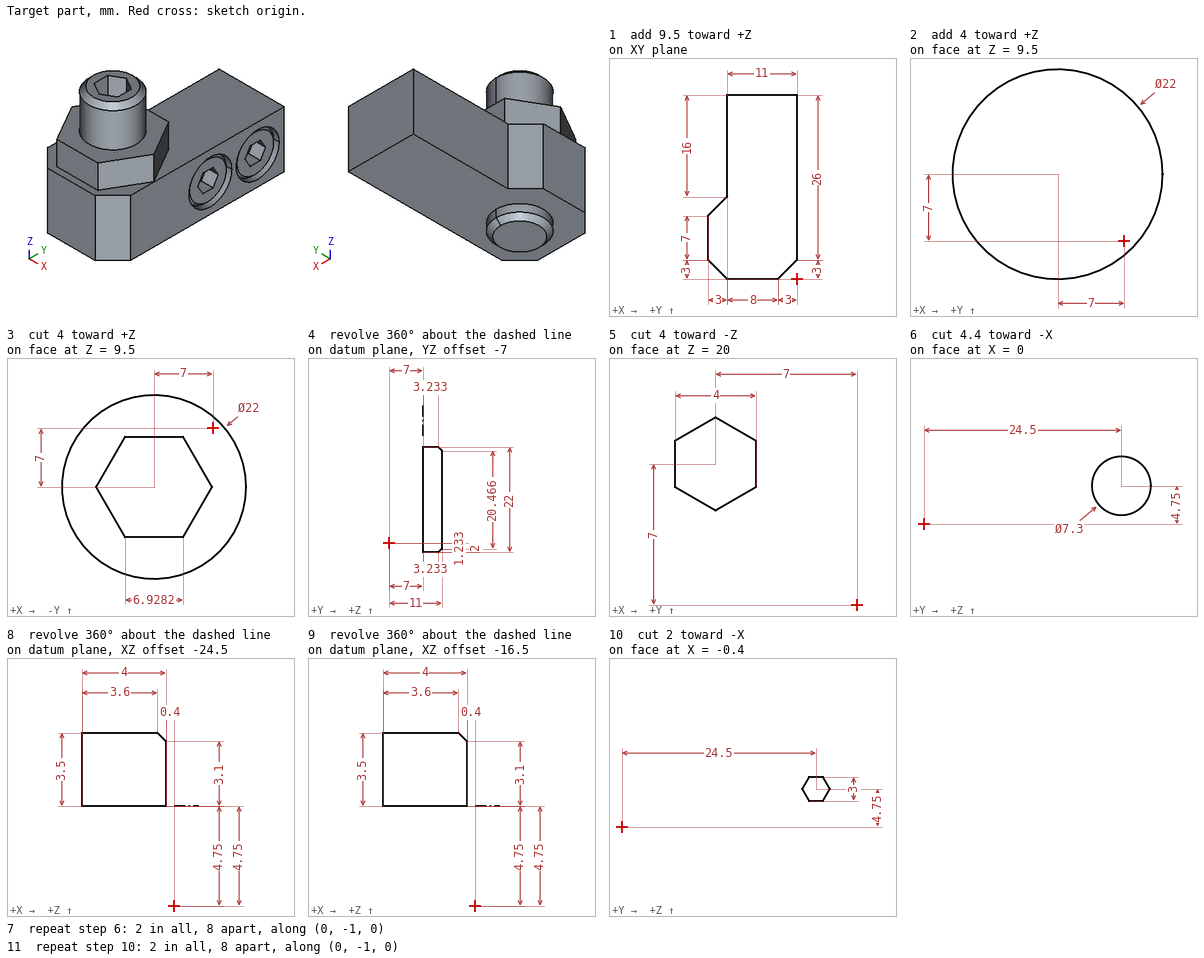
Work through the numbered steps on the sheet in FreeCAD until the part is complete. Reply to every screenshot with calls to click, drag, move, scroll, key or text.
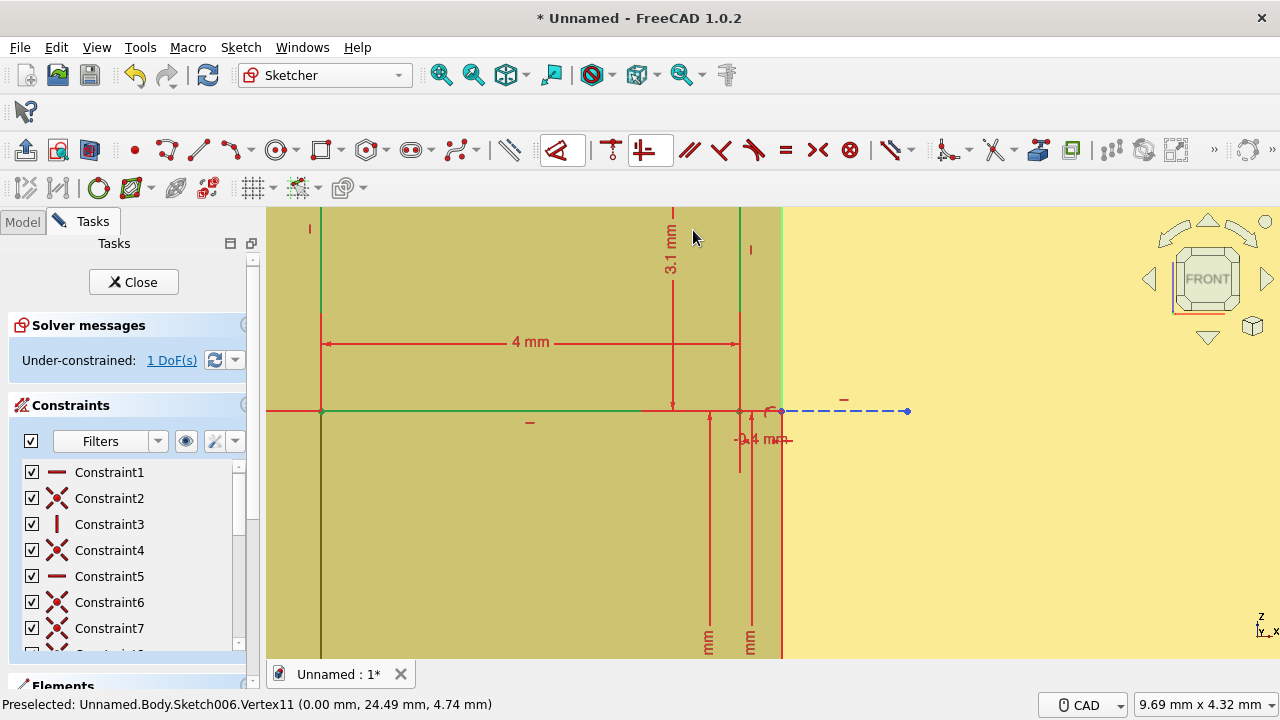
click(134, 282)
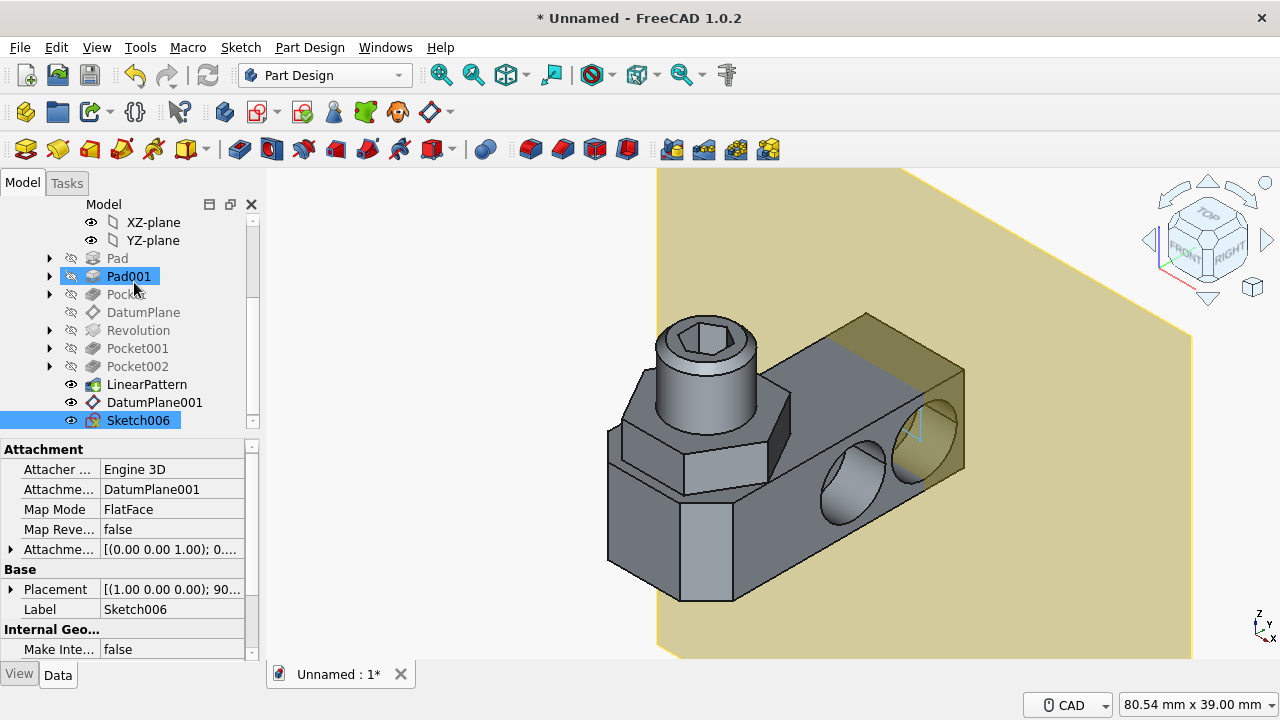
click(58, 150)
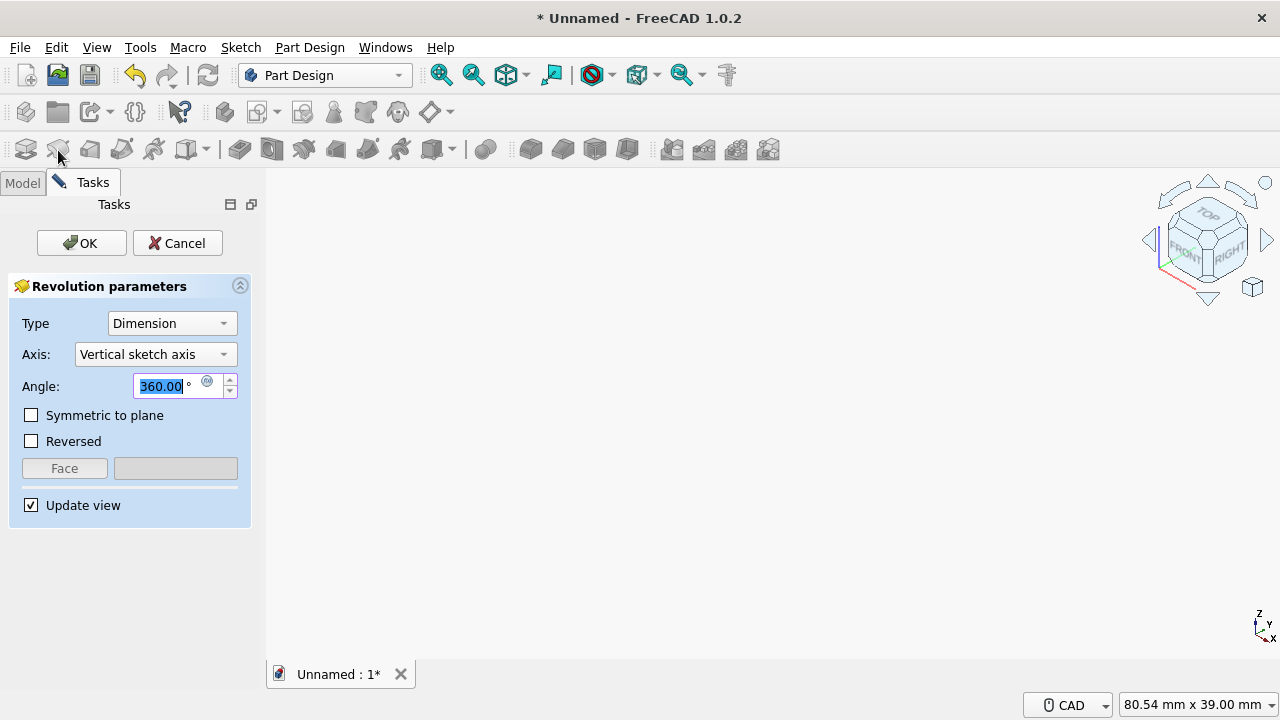
click(156, 354)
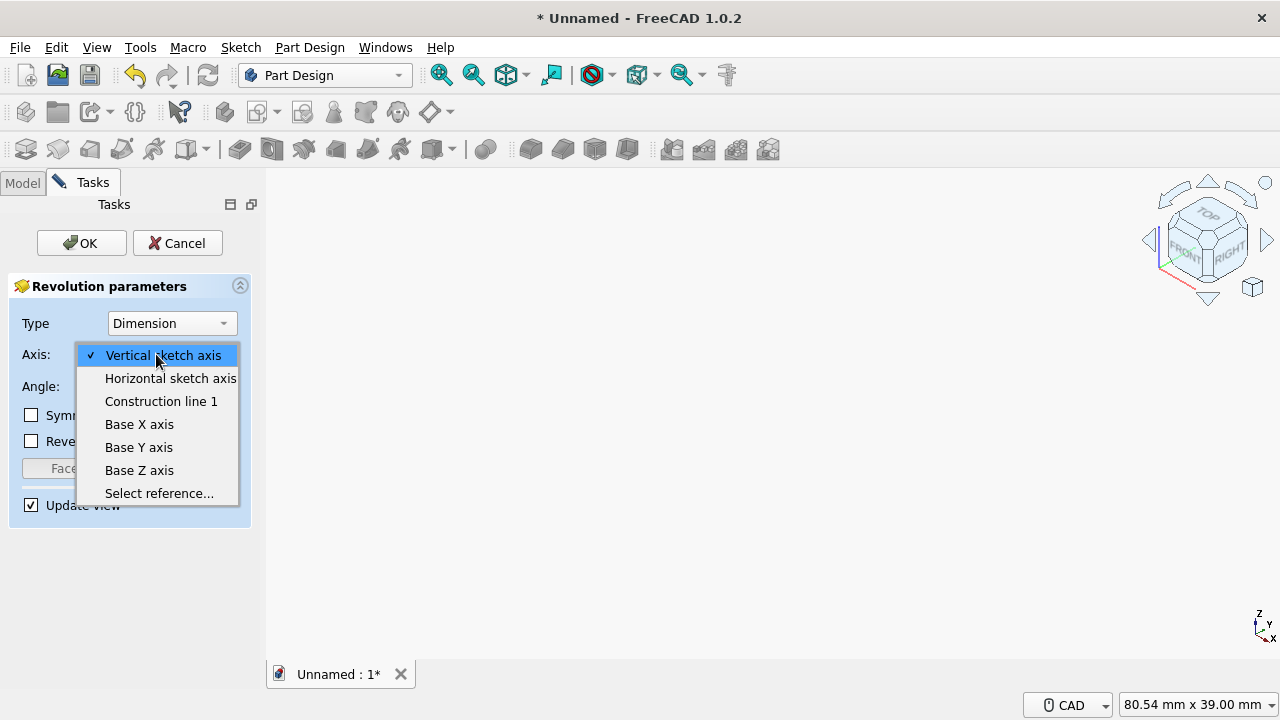
click(156, 402)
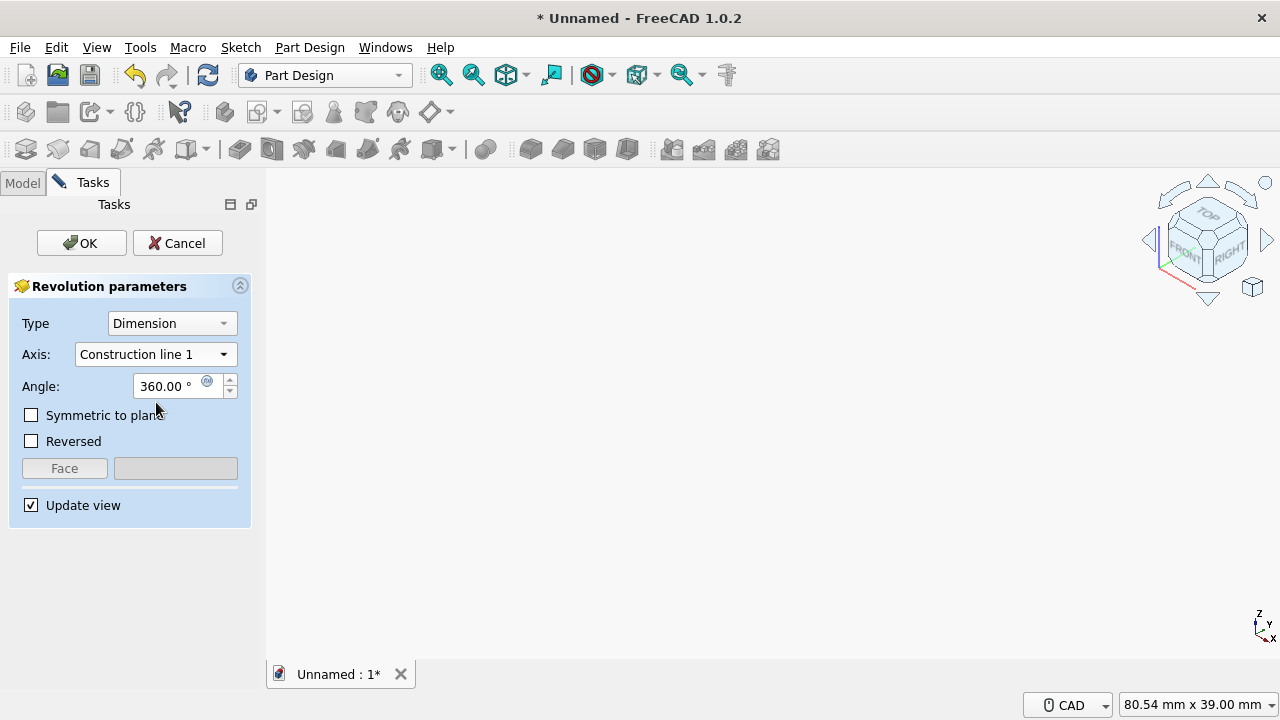
click(82, 243)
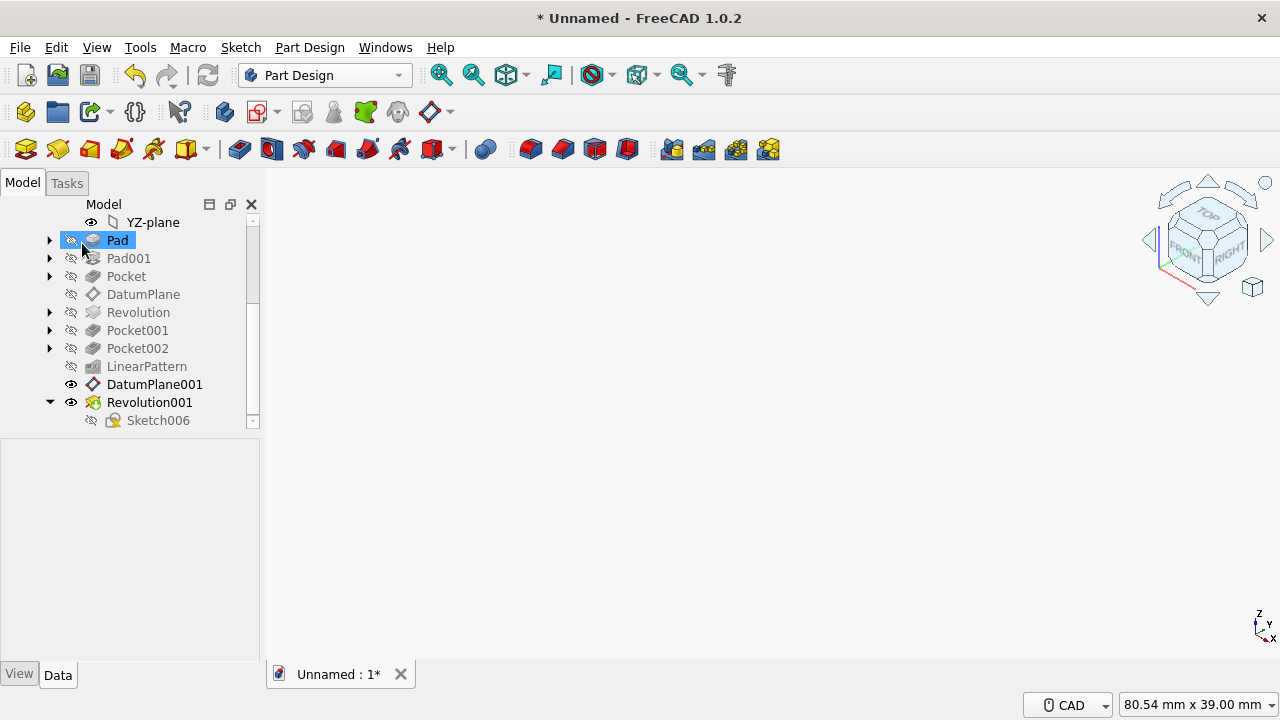
click(116, 384)
key(space)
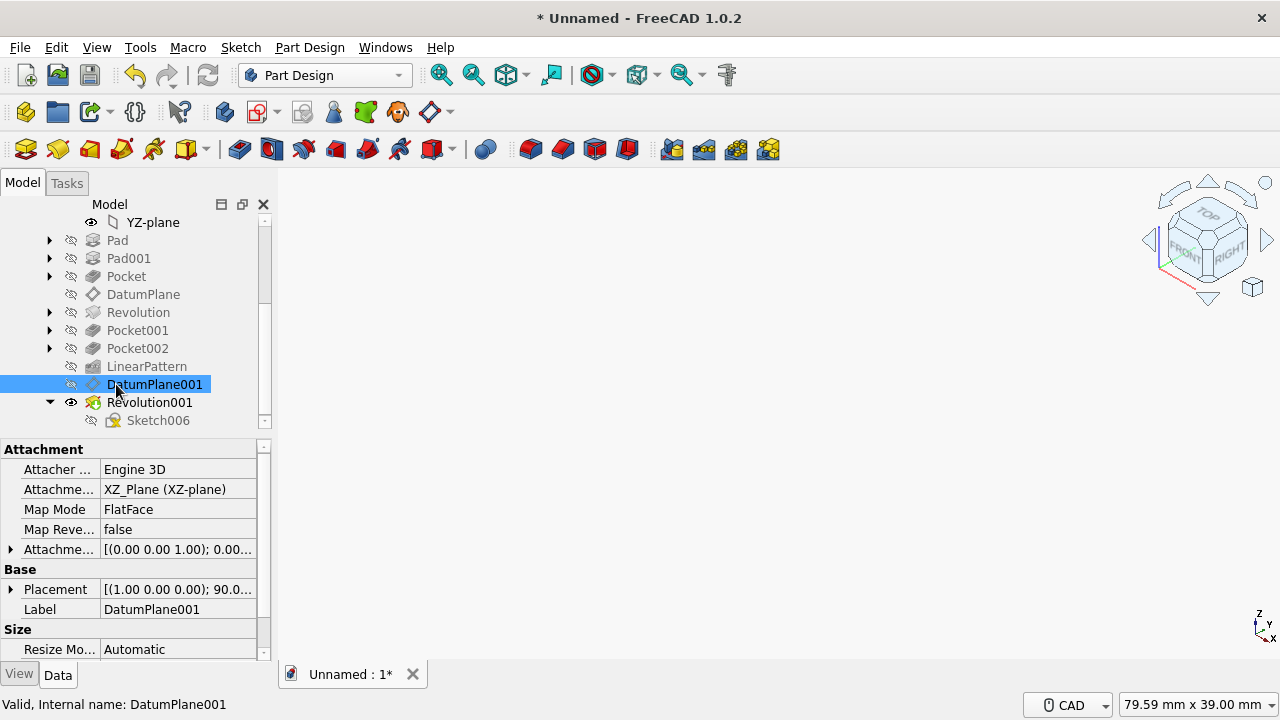
key(v)
key(f)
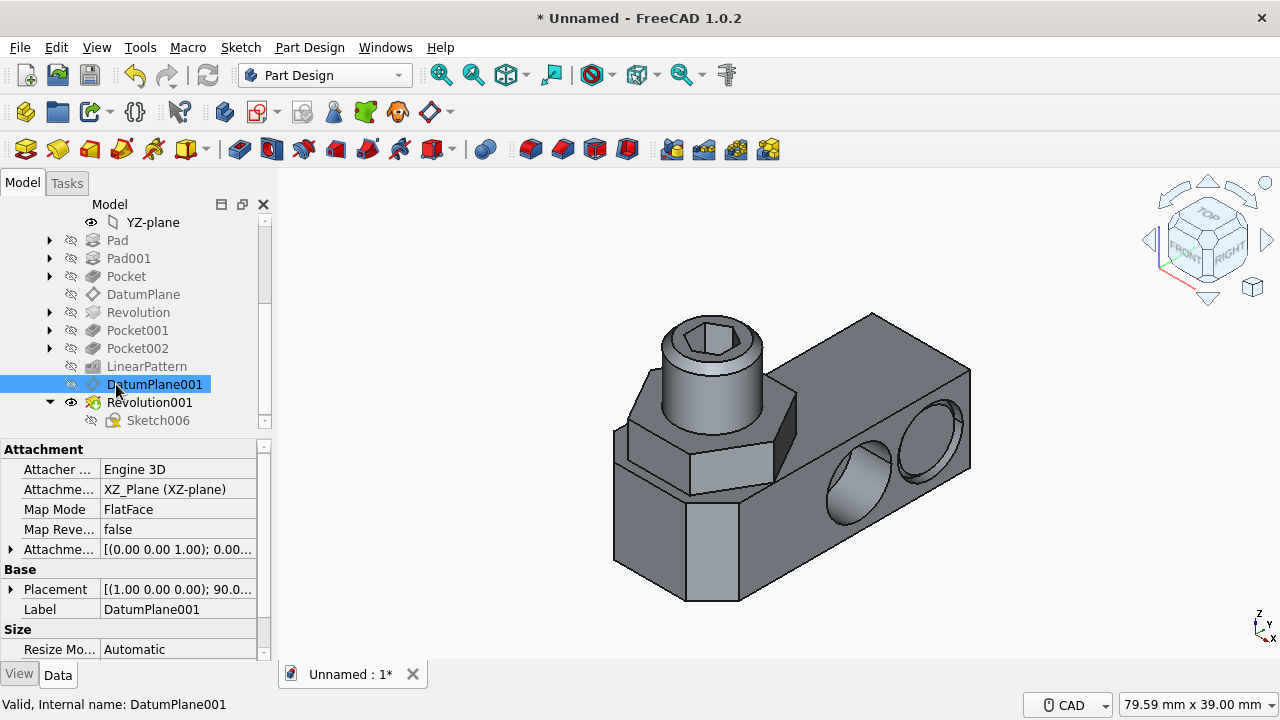
scroll(160, 326, down, 3)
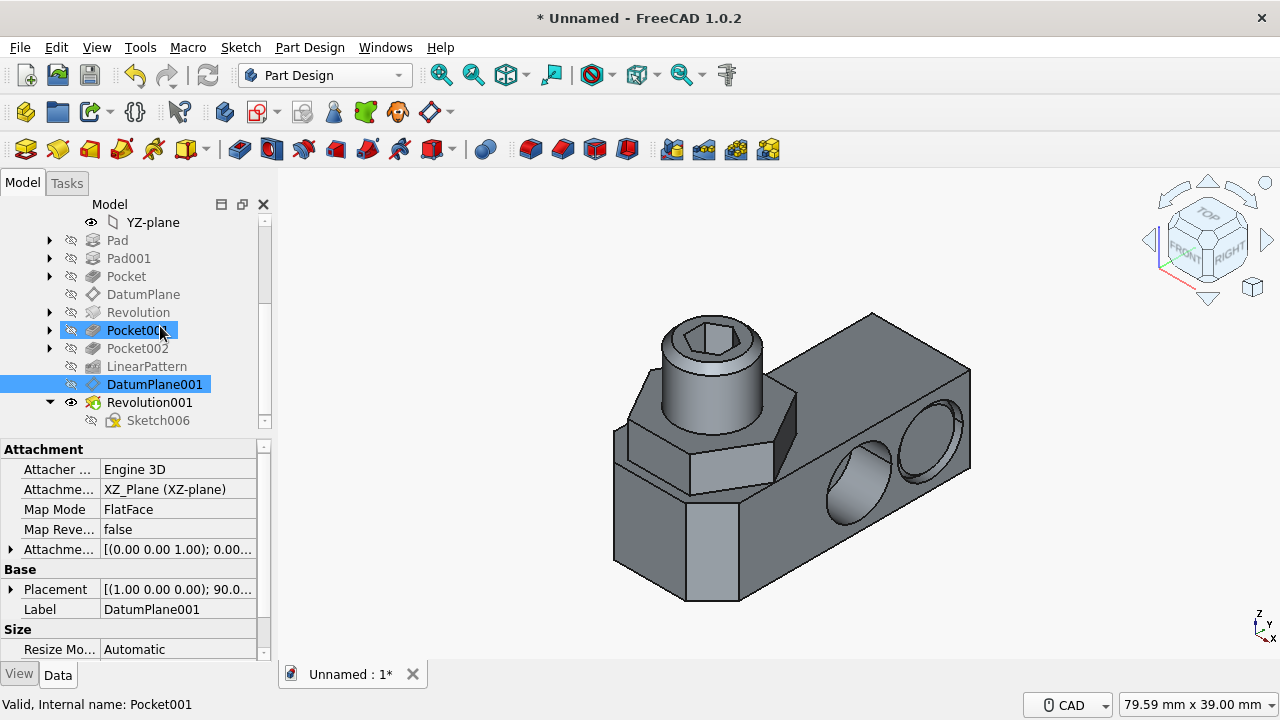
scroll(160, 326, up, 15)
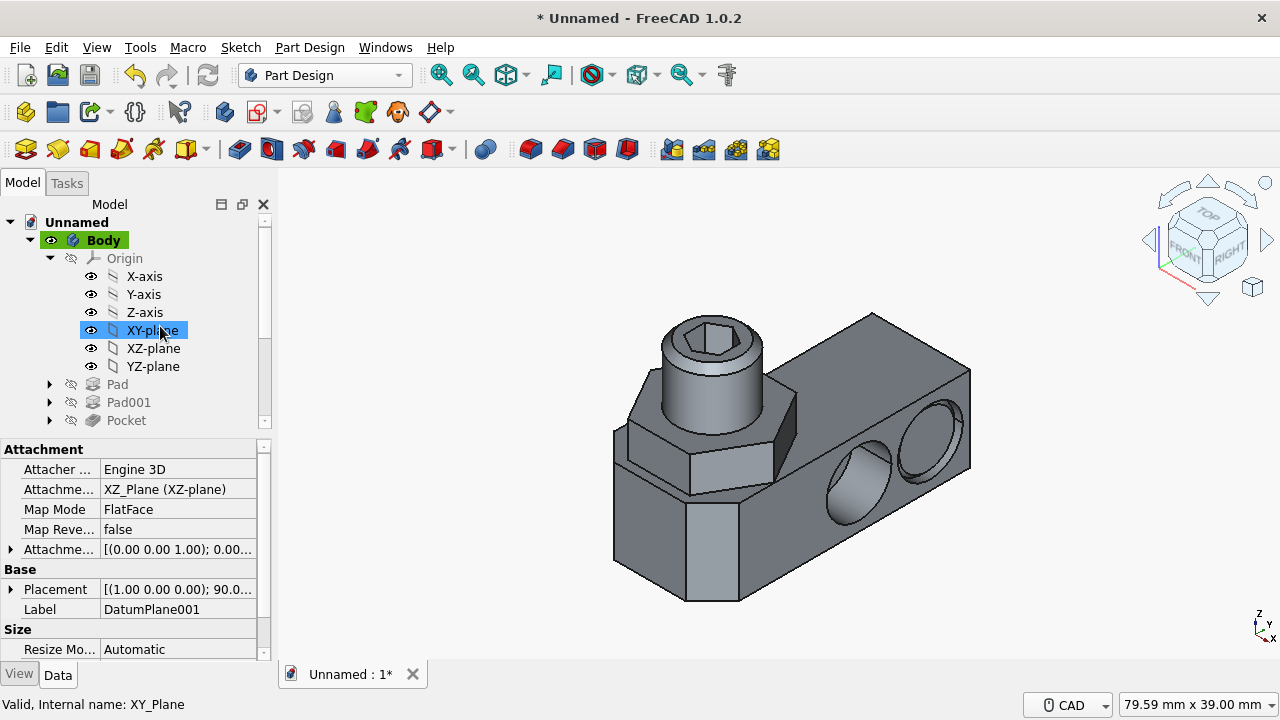
click(136, 348)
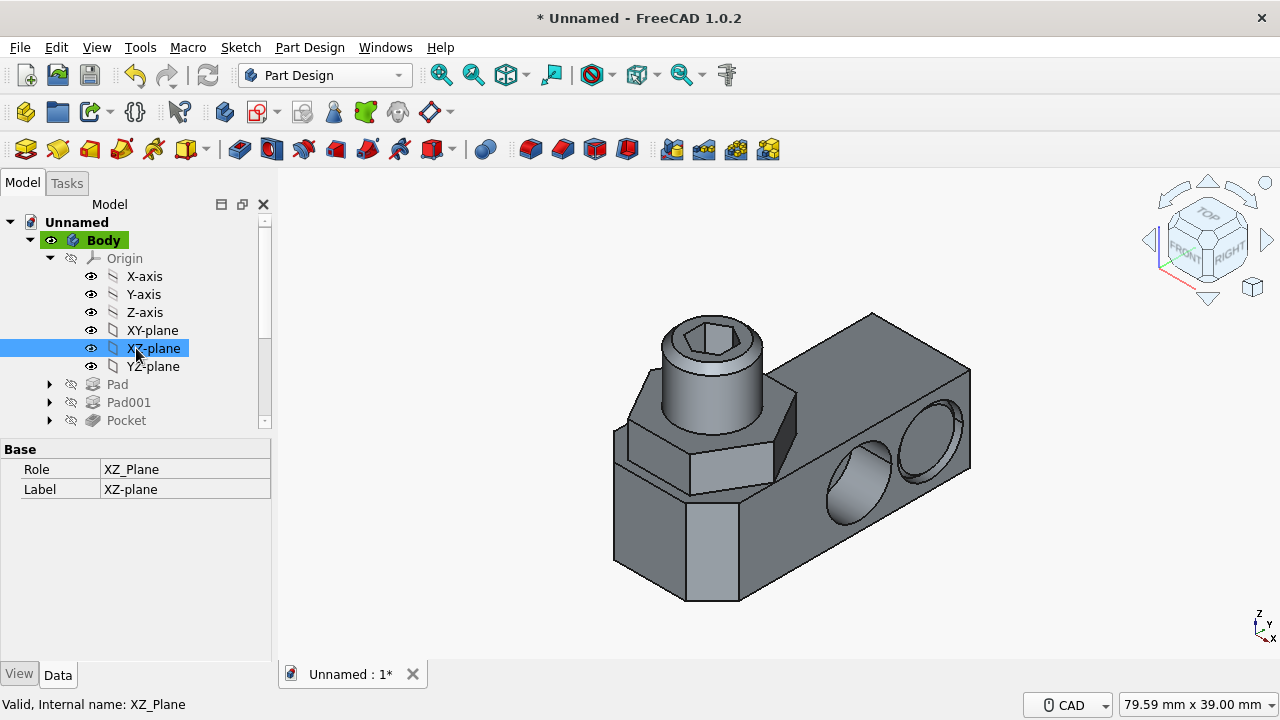
click(430, 112)